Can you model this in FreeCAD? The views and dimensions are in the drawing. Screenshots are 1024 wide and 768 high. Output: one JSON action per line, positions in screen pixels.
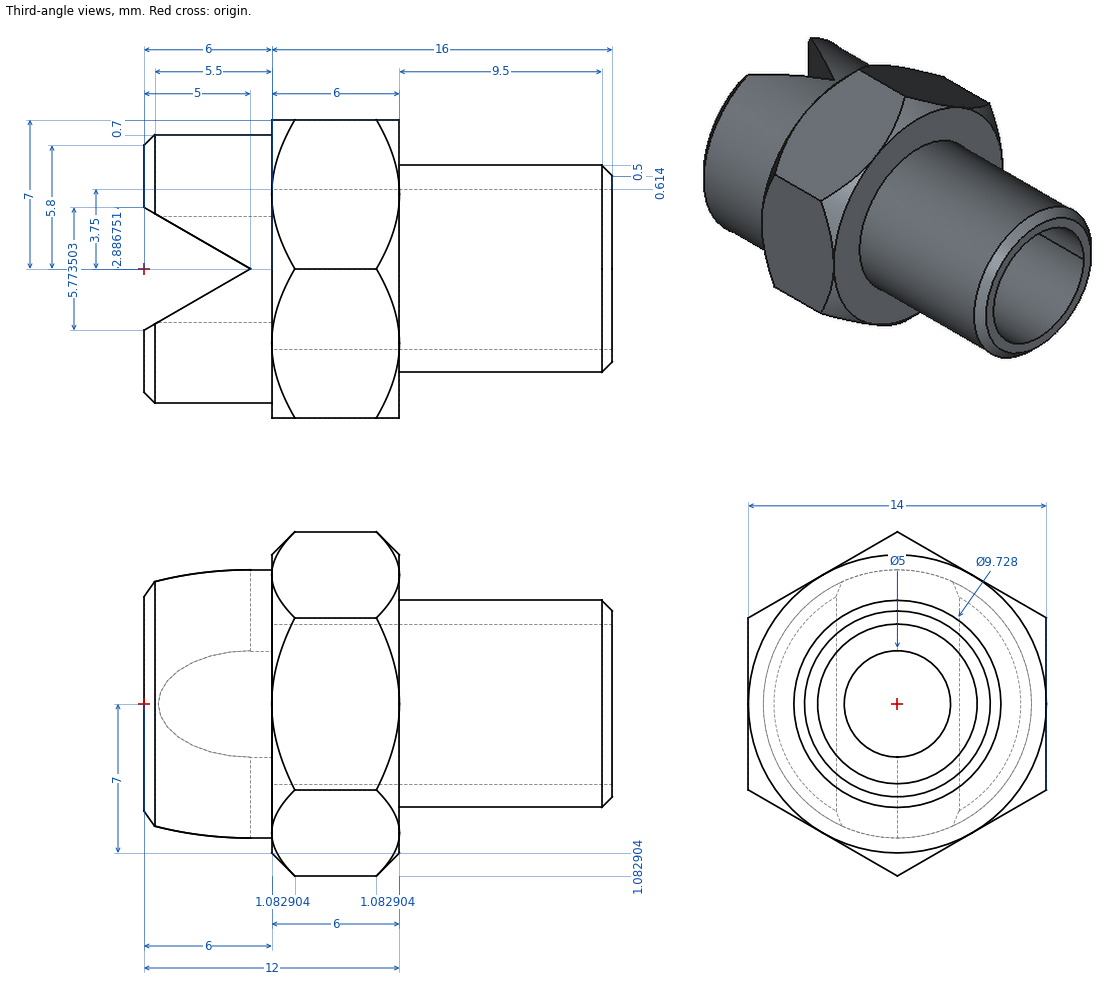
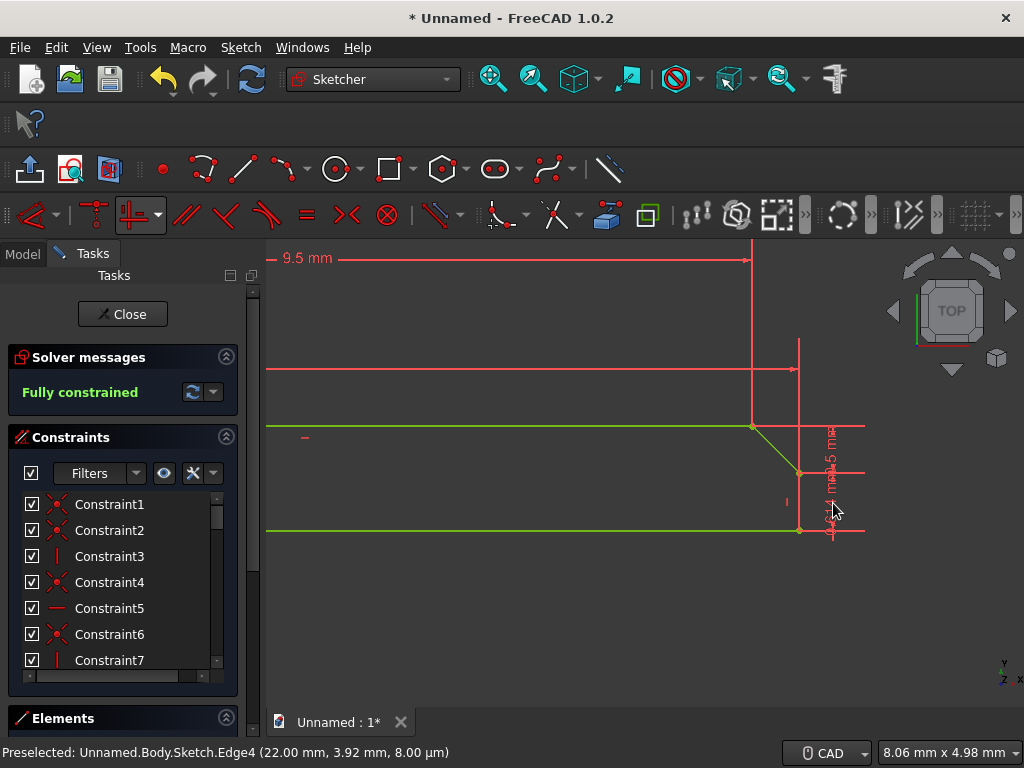
{"action": "left_click", "coordinate": [123, 314]}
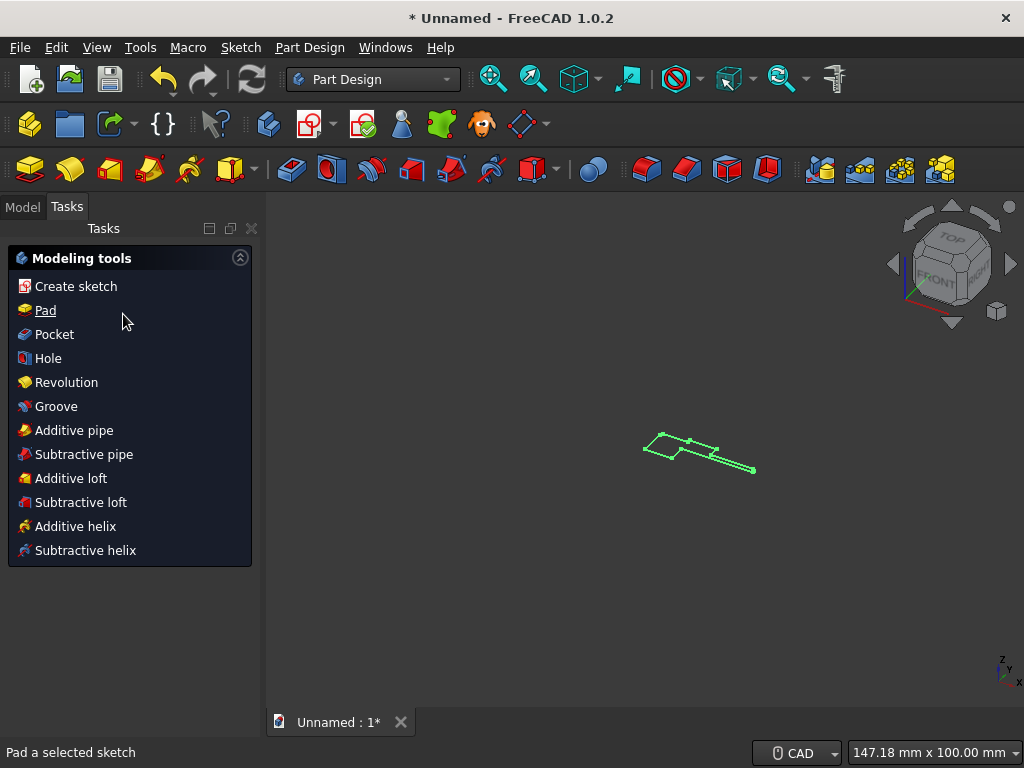
{"action": "left_click", "coordinate": [70, 170]}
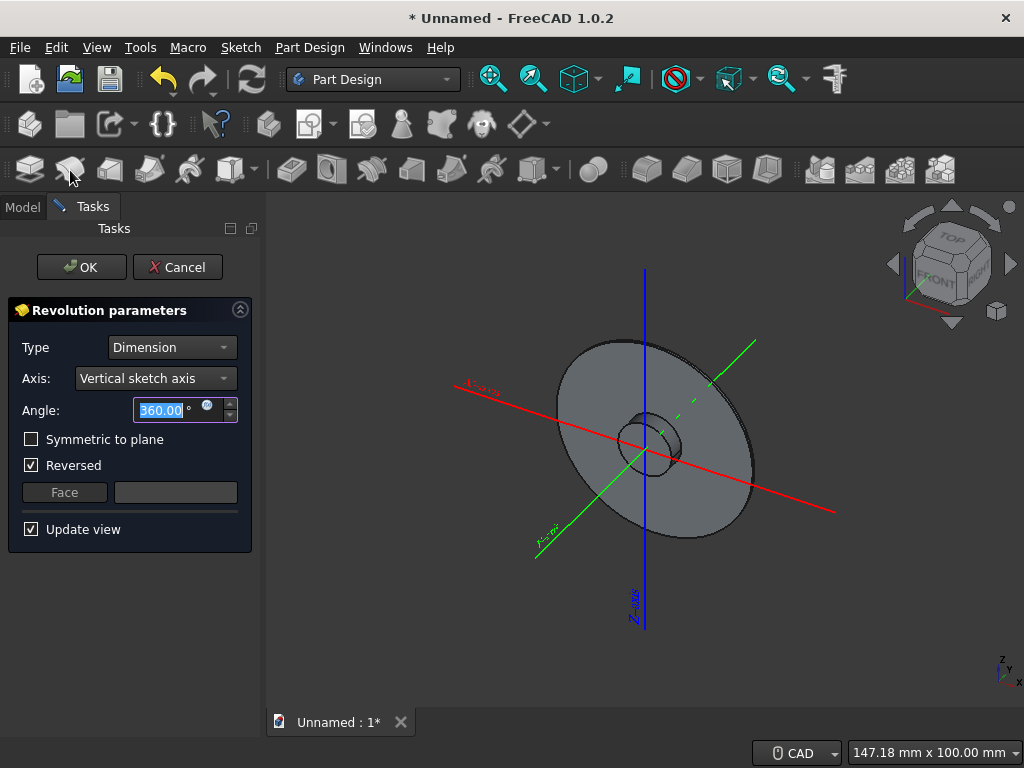
{"action": "left_click", "coordinate": [156, 378]}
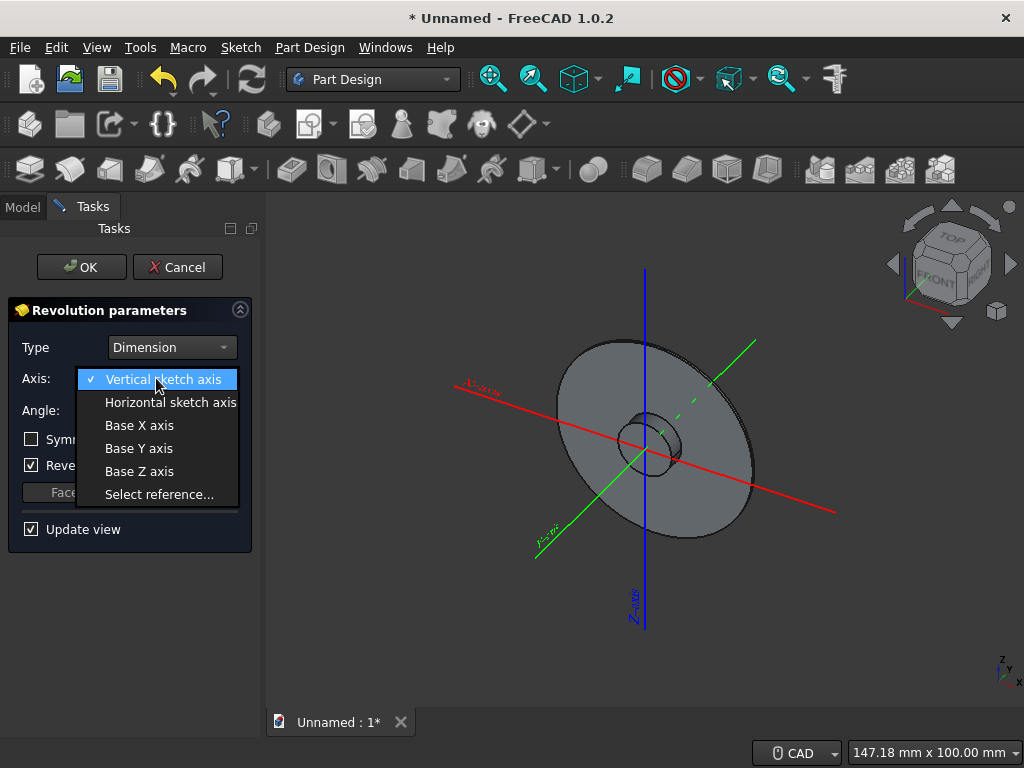
{"action": "left_click", "coordinate": [156, 402]}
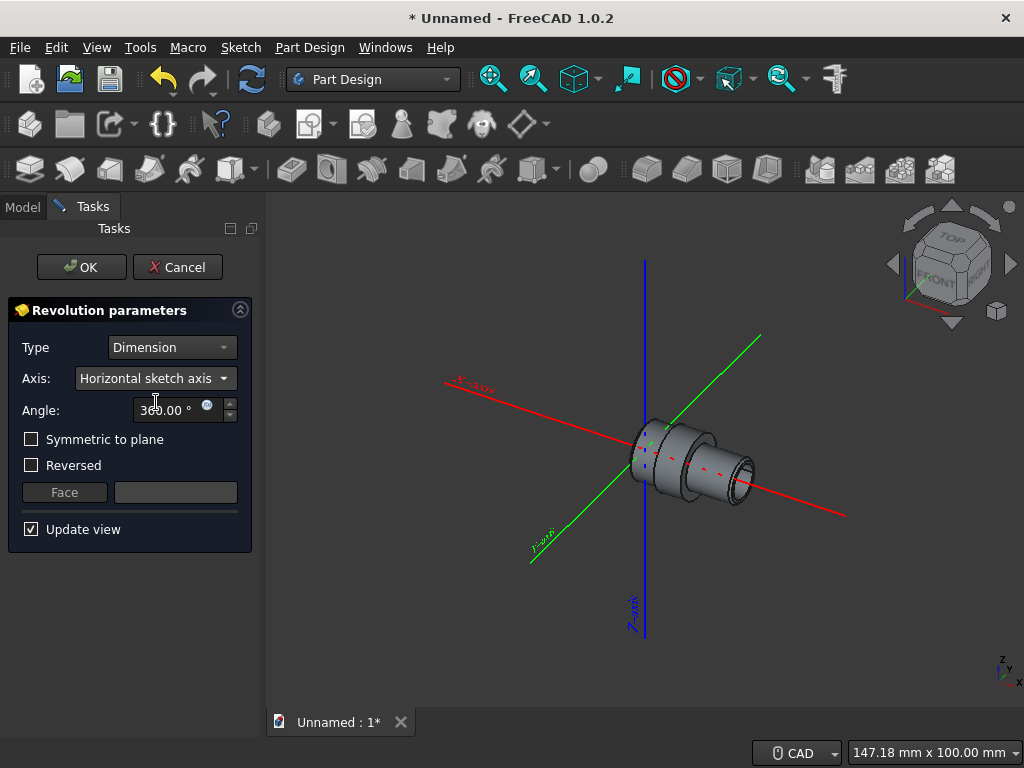
{"action": "left_click", "coordinate": [82, 267]}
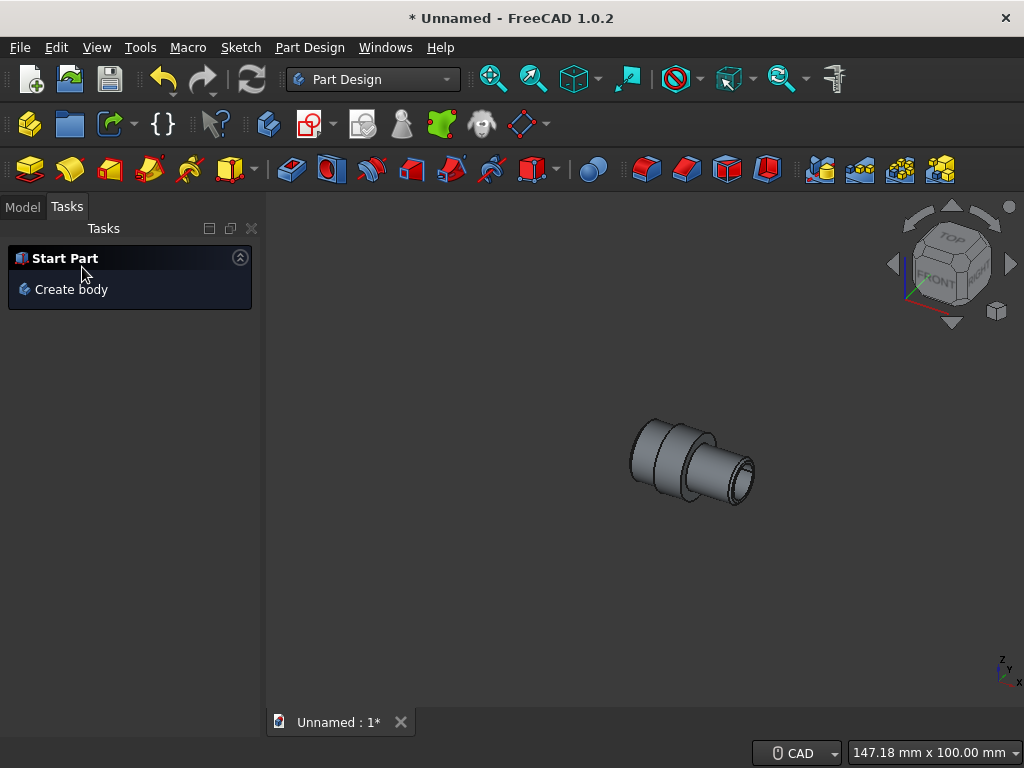
{"action": "left_click", "coordinate": [494, 80]}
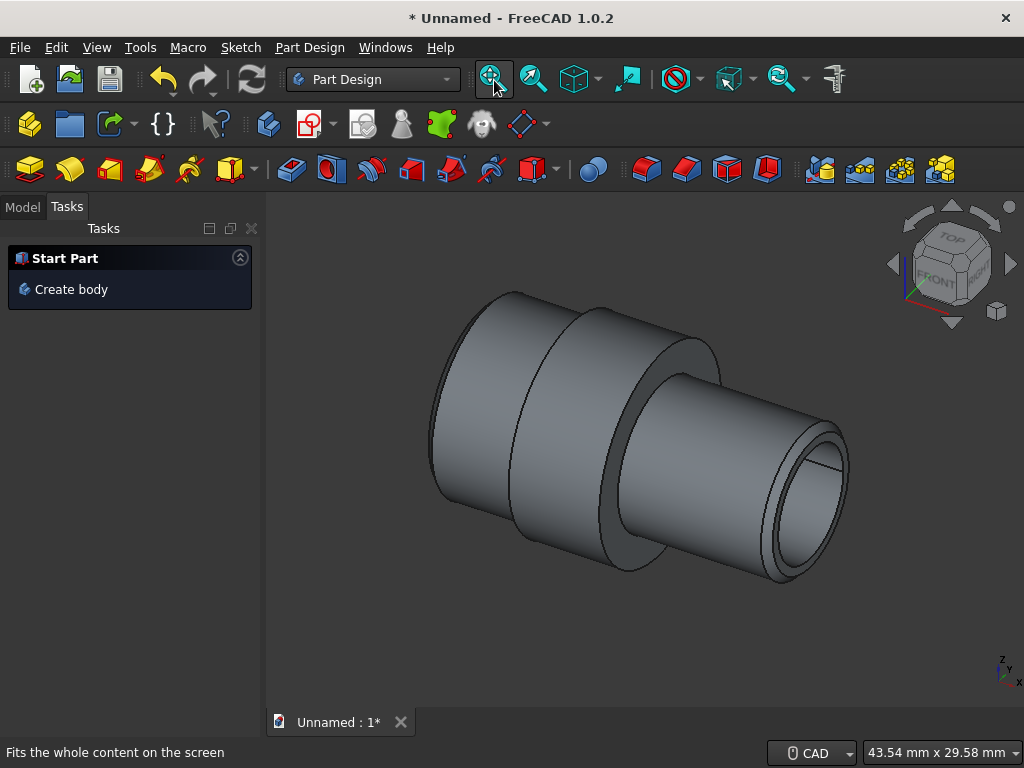
{"action": "left_click", "coordinate": [660, 368]}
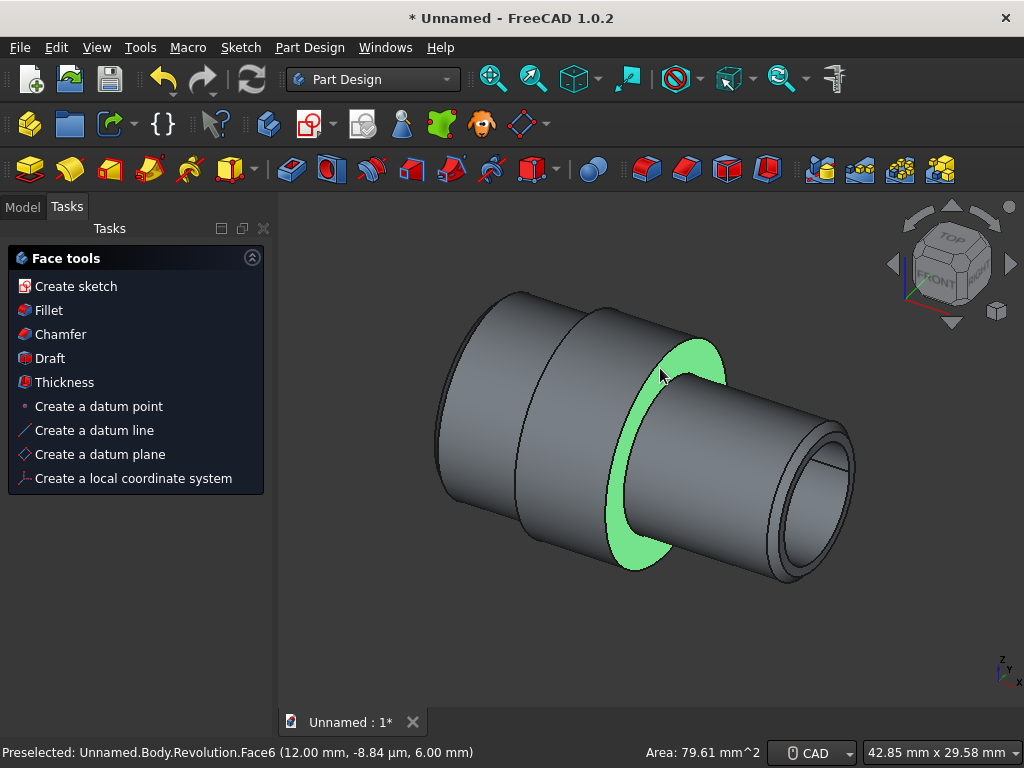
{"action": "left_click", "coordinate": [310, 124]}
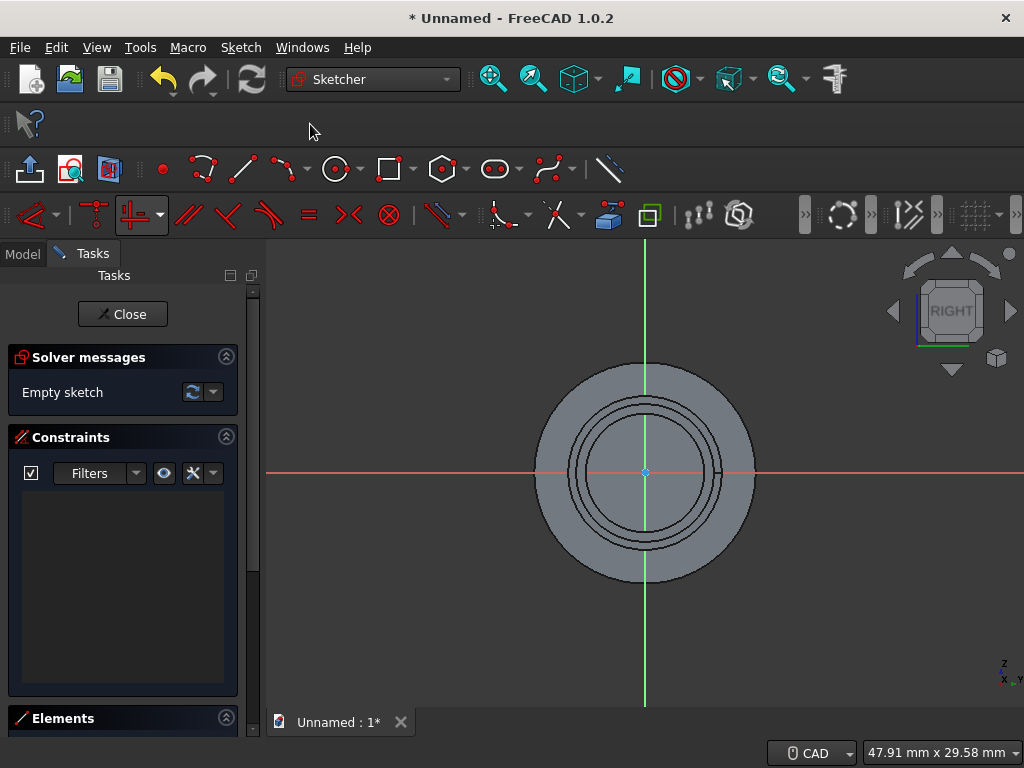
{"action": "left_click", "coordinate": [110, 170]}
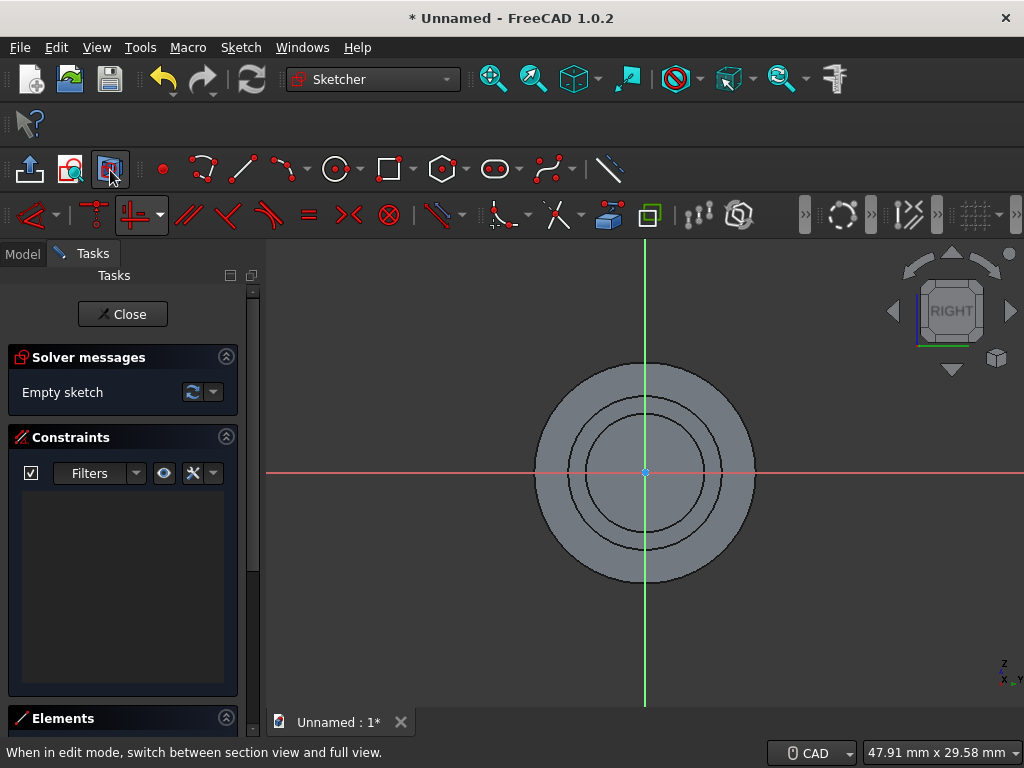
{"action": "left_click", "coordinate": [442, 170]}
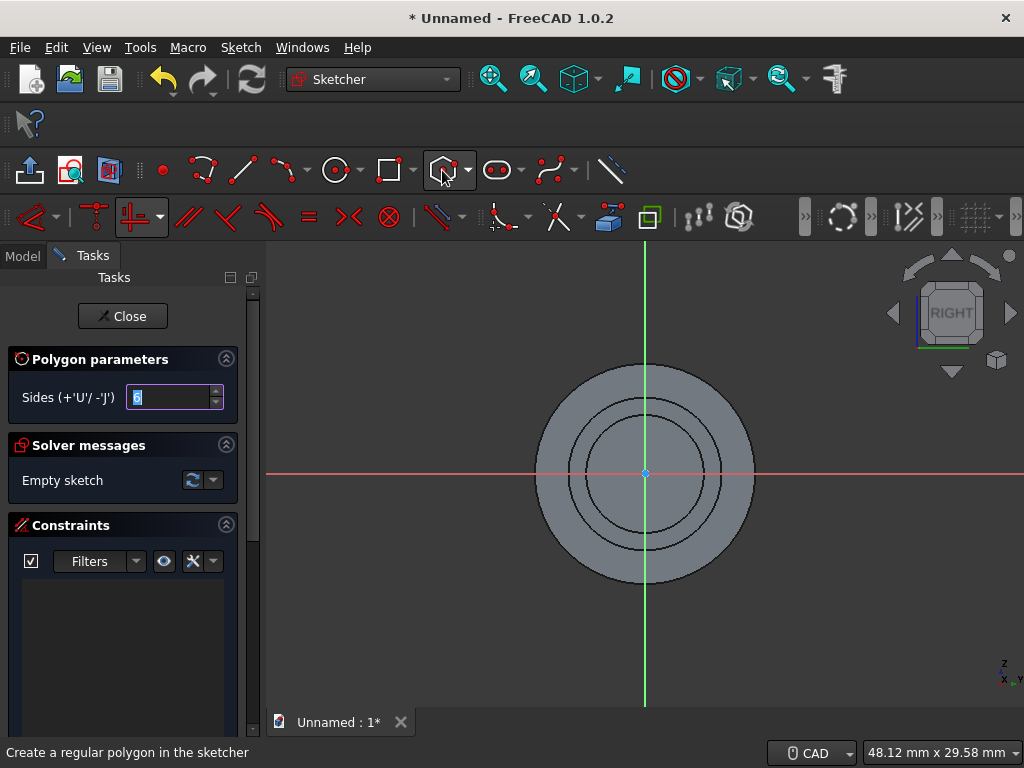
{"action": "left_click", "coordinate": [645, 474]}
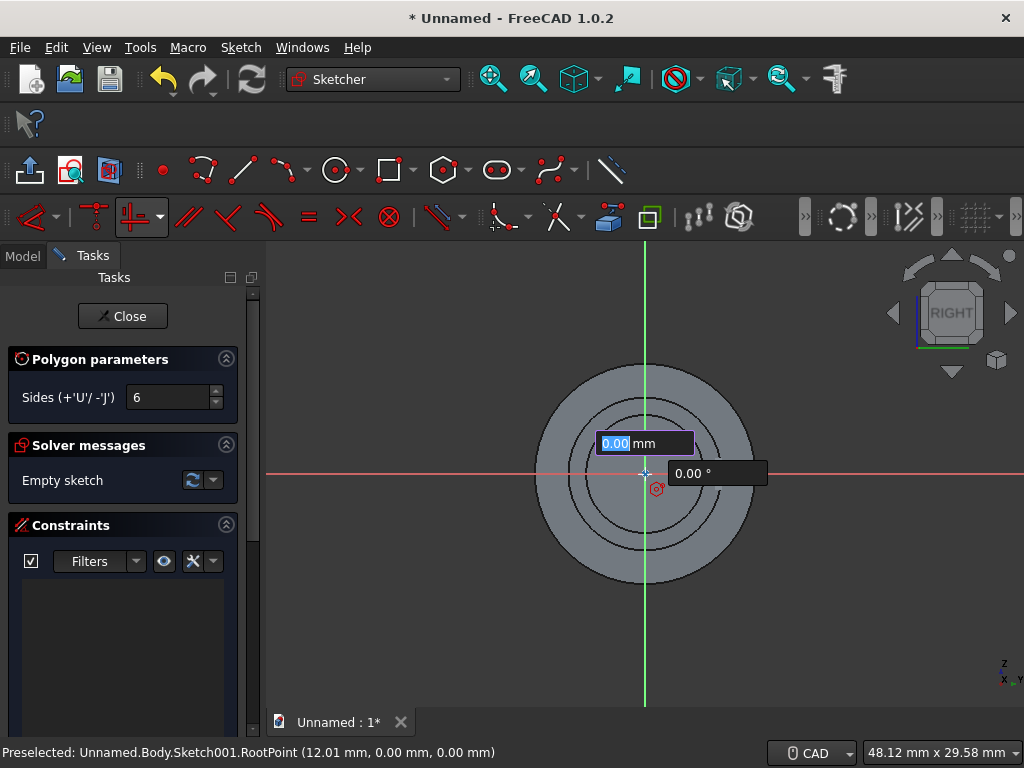
{"action": "left_click", "coordinate": [645, 601]}
{"action": "right_click", "coordinate": [645, 601]}